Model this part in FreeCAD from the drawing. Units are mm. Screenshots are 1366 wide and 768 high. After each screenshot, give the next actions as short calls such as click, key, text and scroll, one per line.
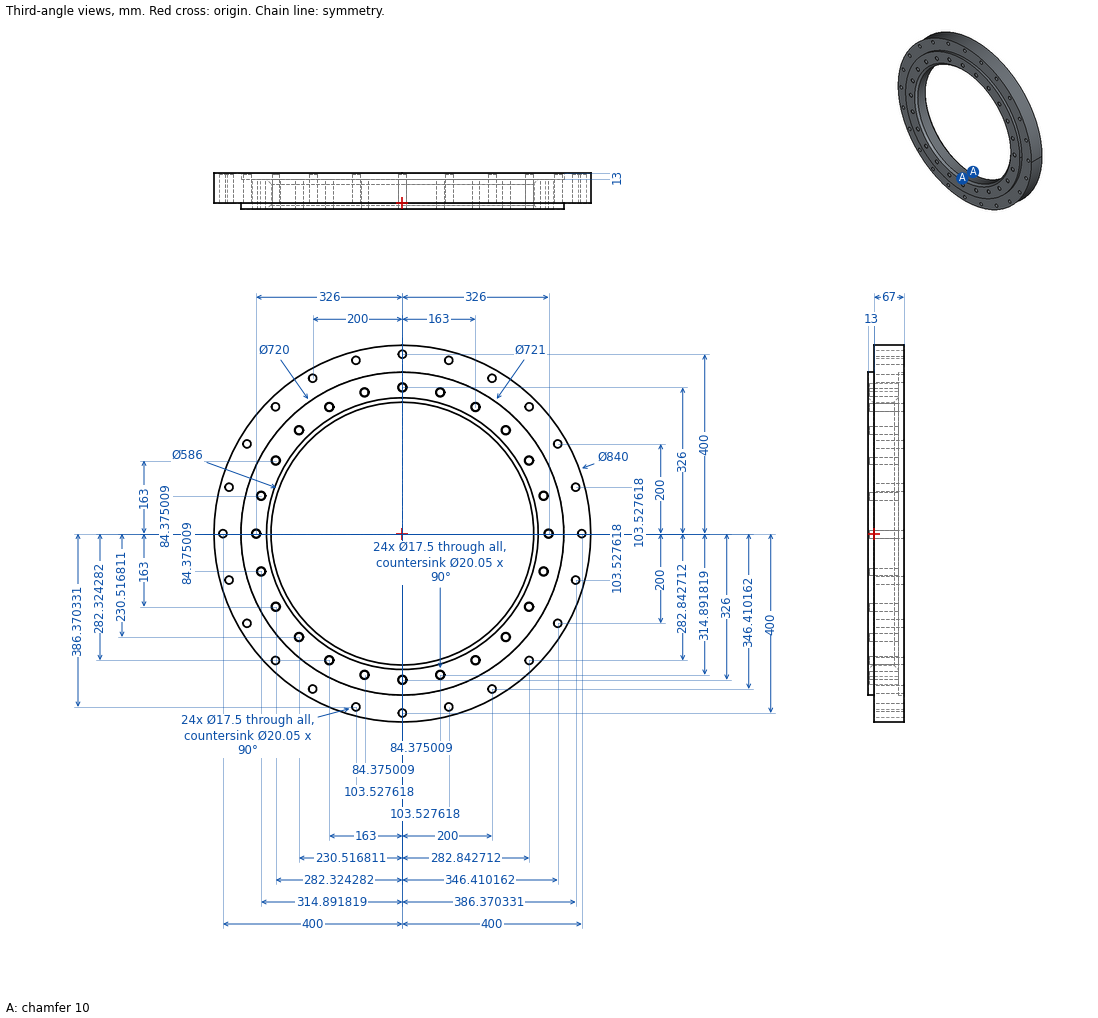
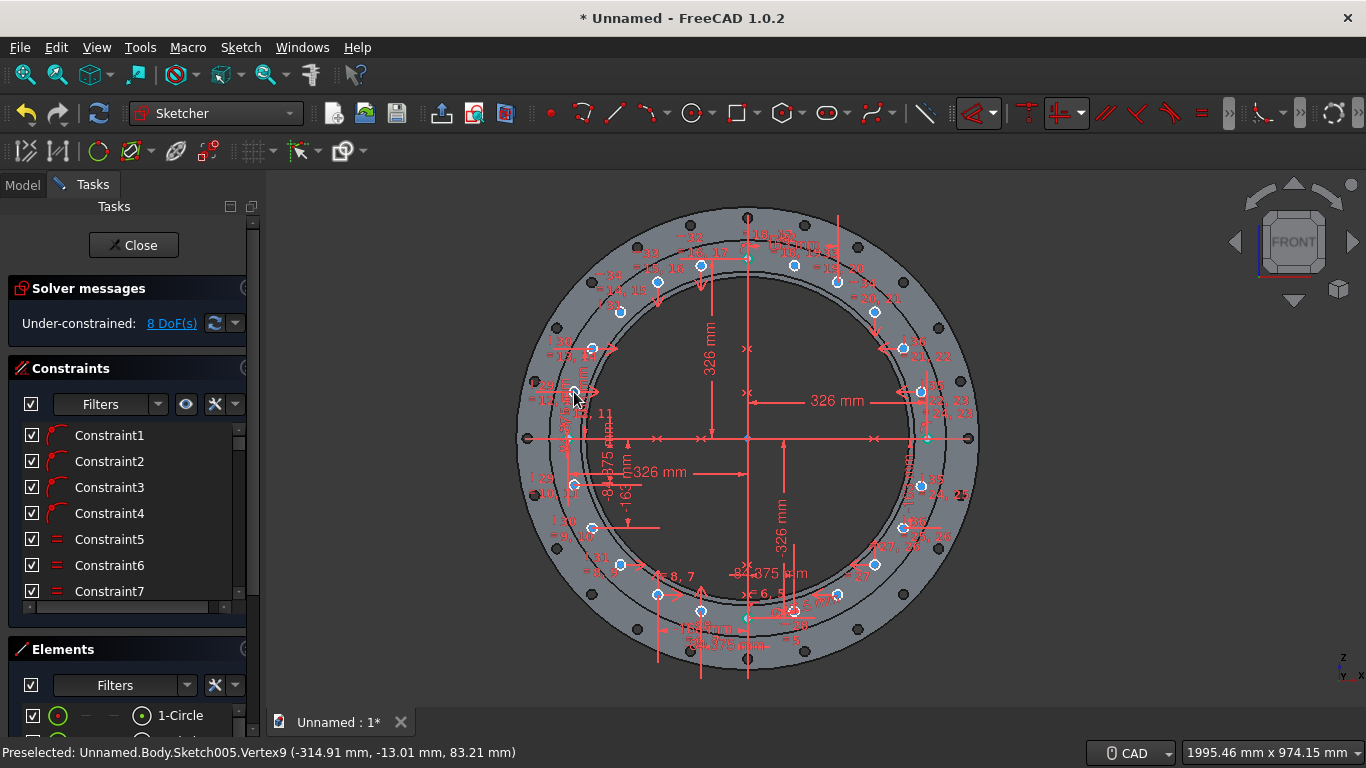
click(795, 266)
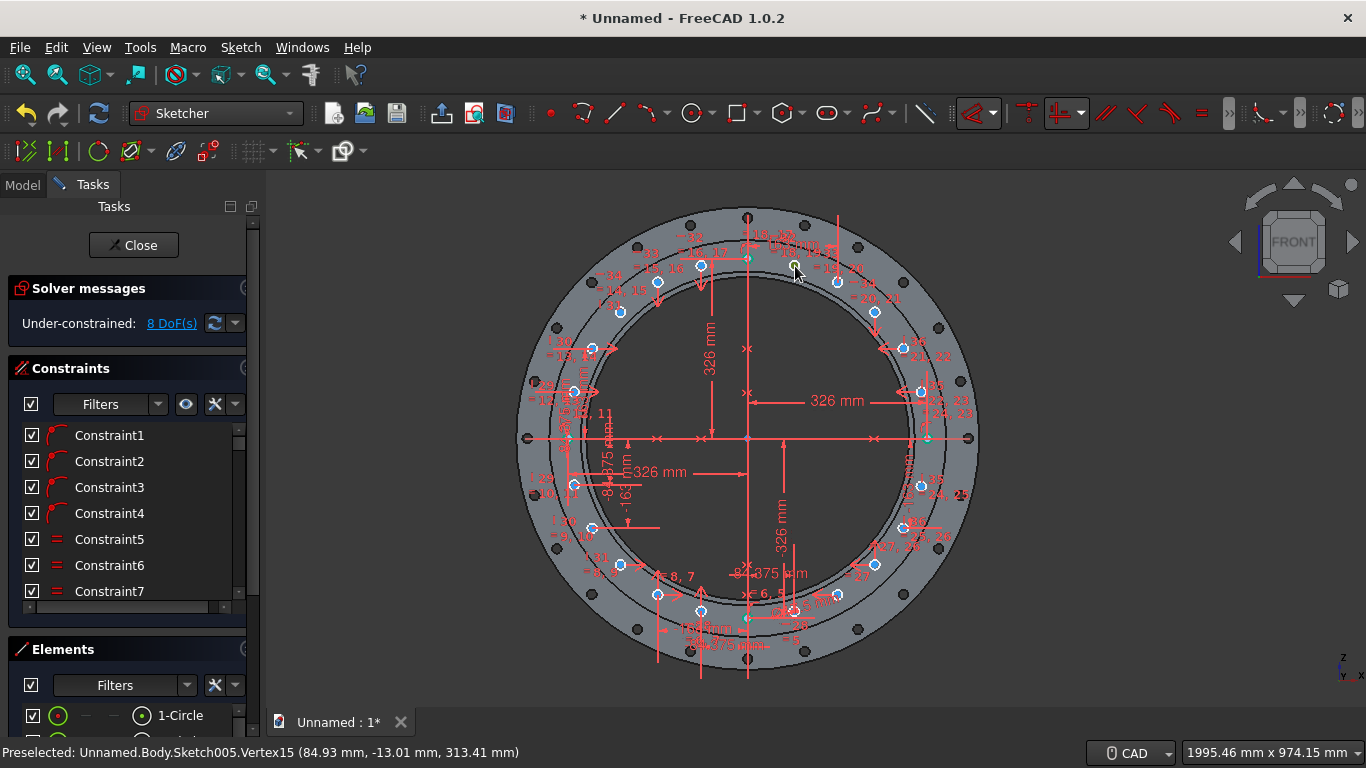
click(996, 114)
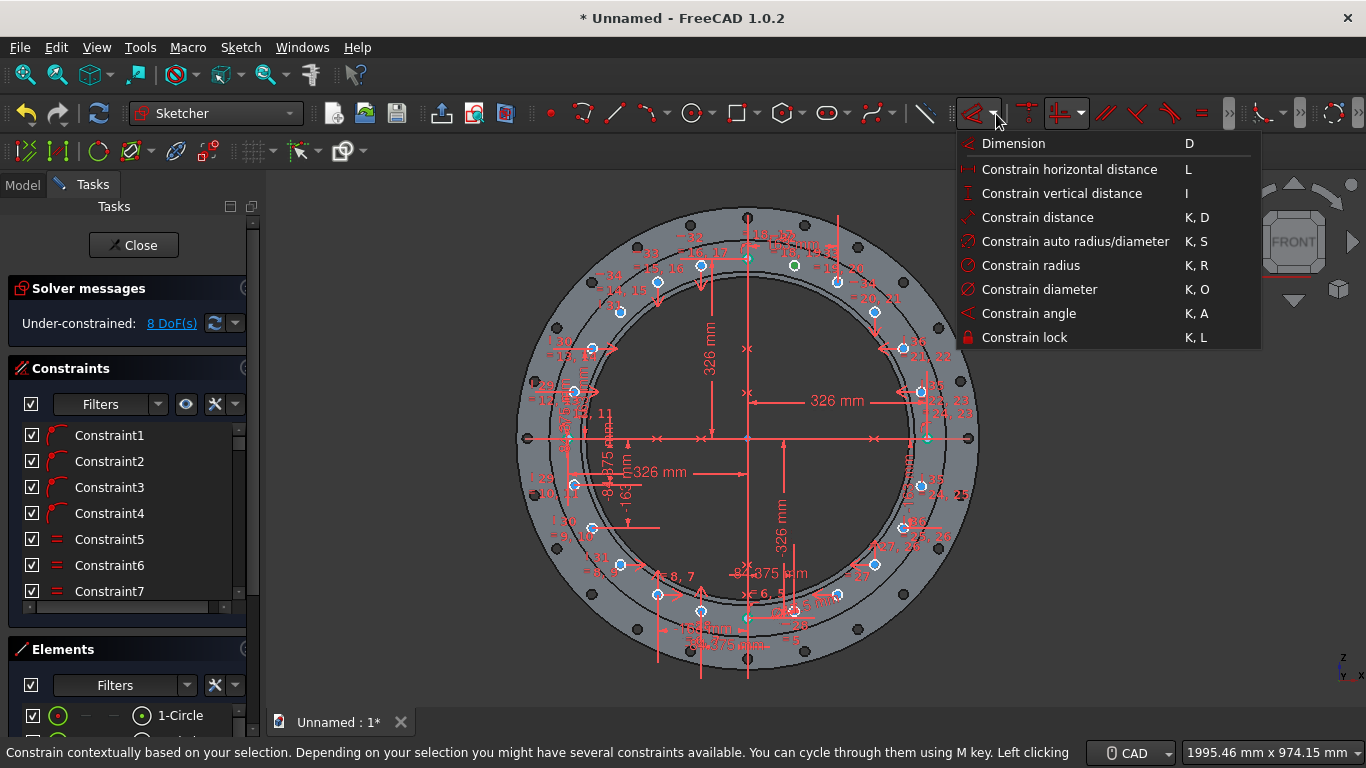
click(1109, 169)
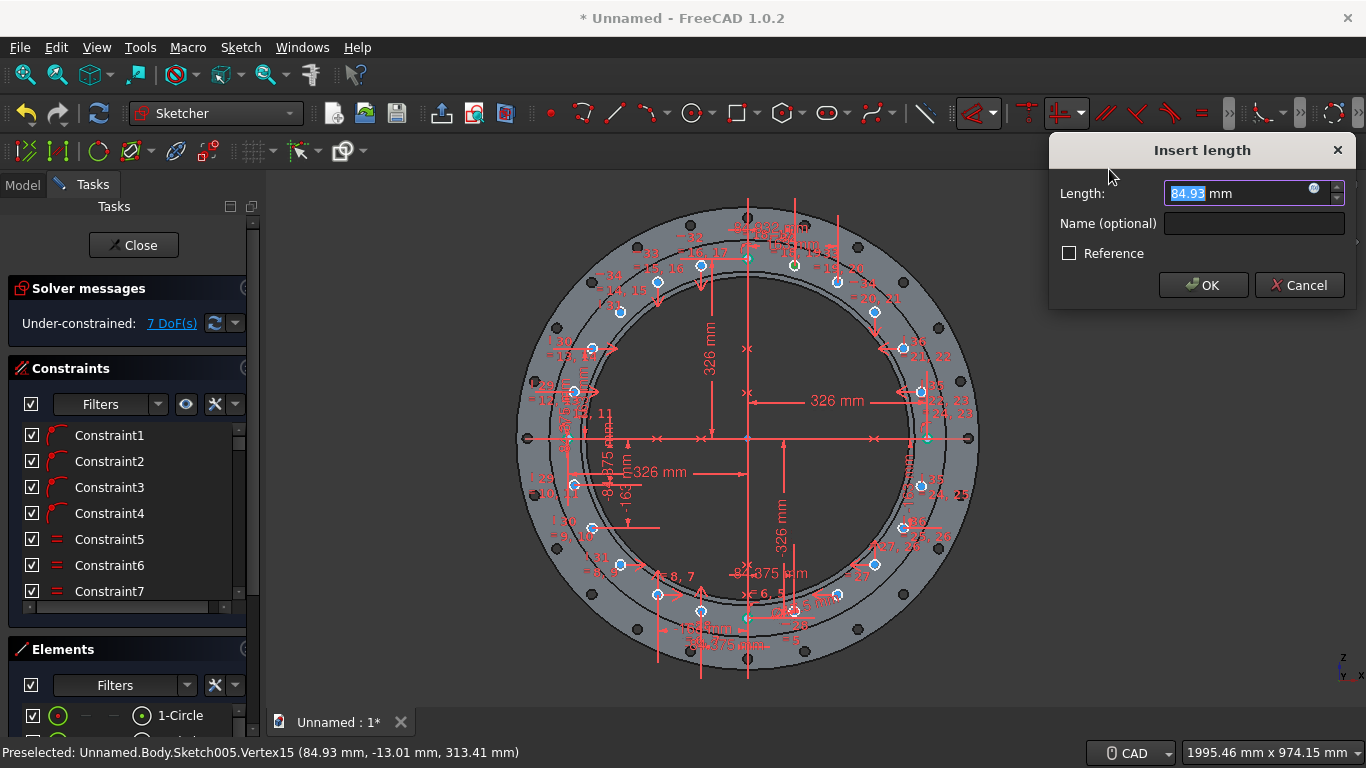
text(84.375009)
key(Return)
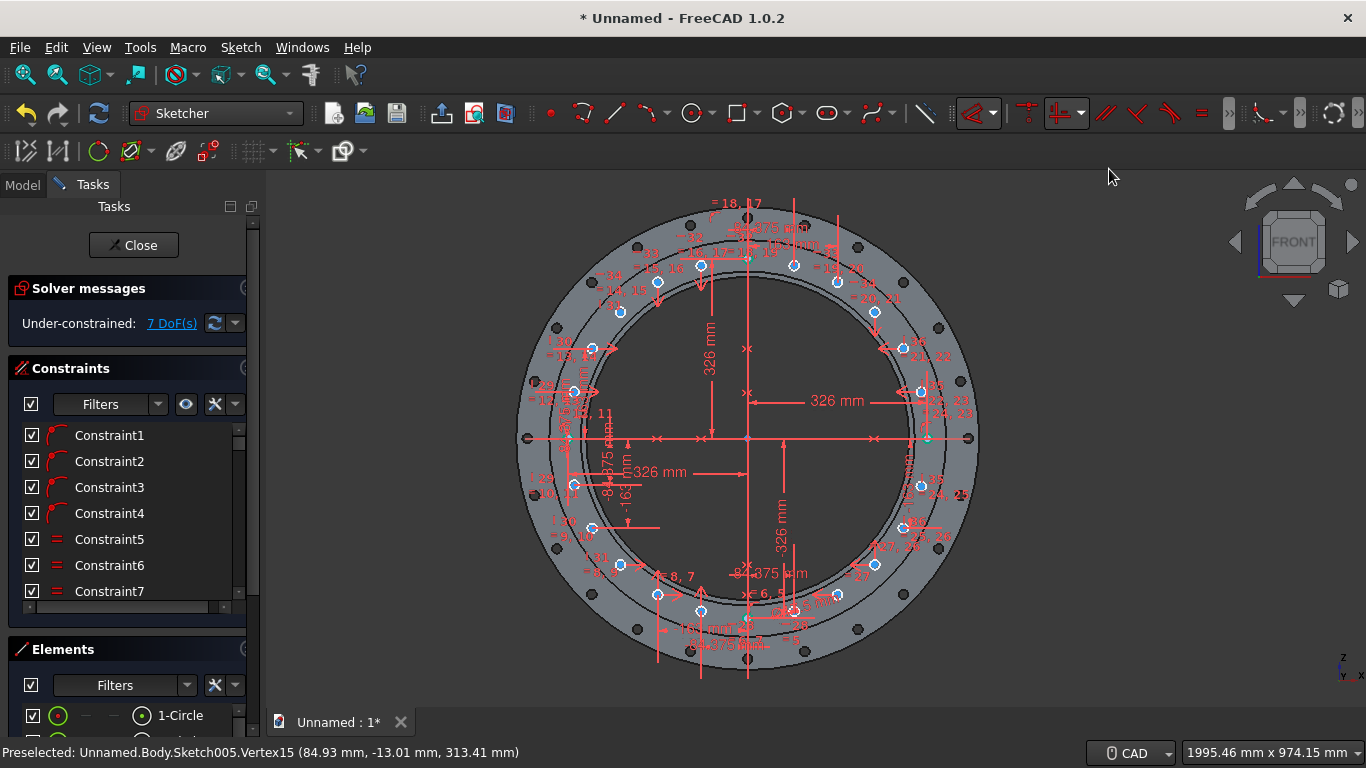
scroll(921, 486, up, 4)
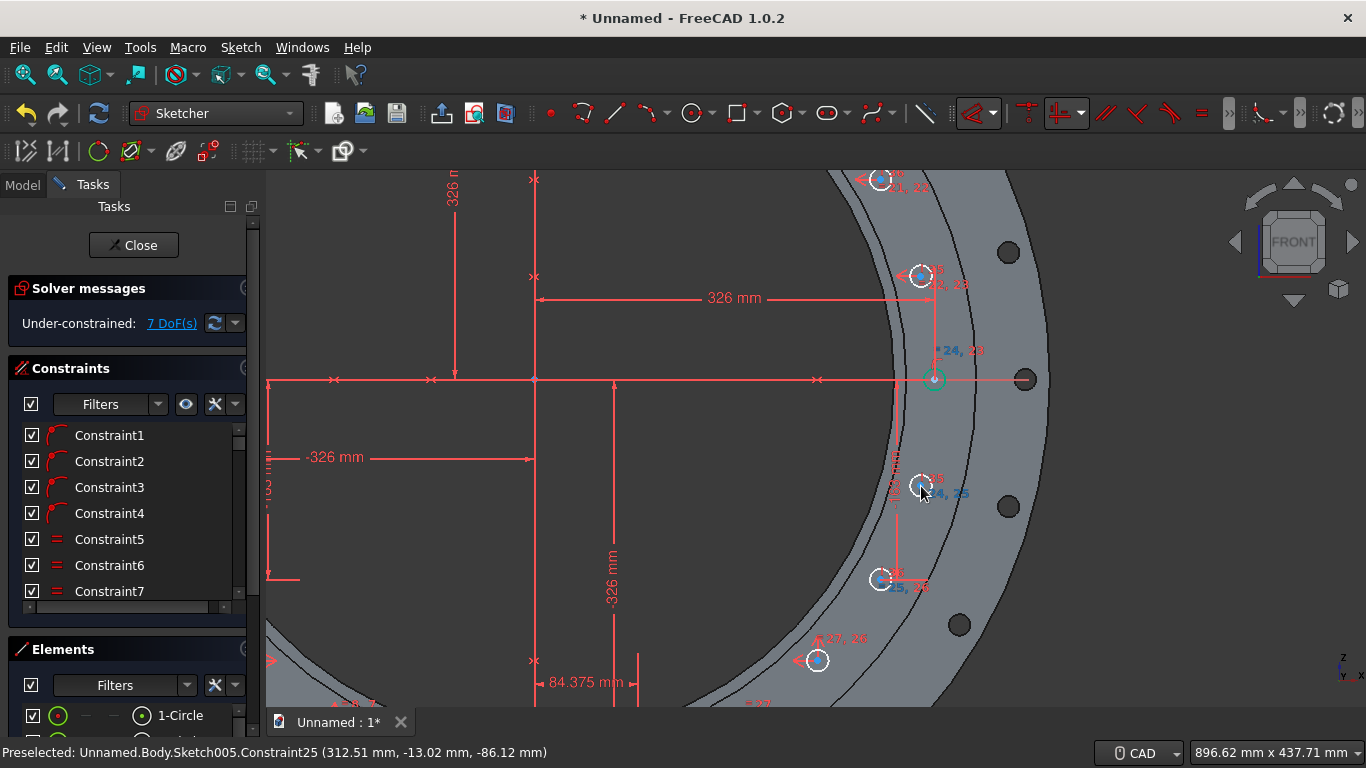
scroll(921, 486, up, 4)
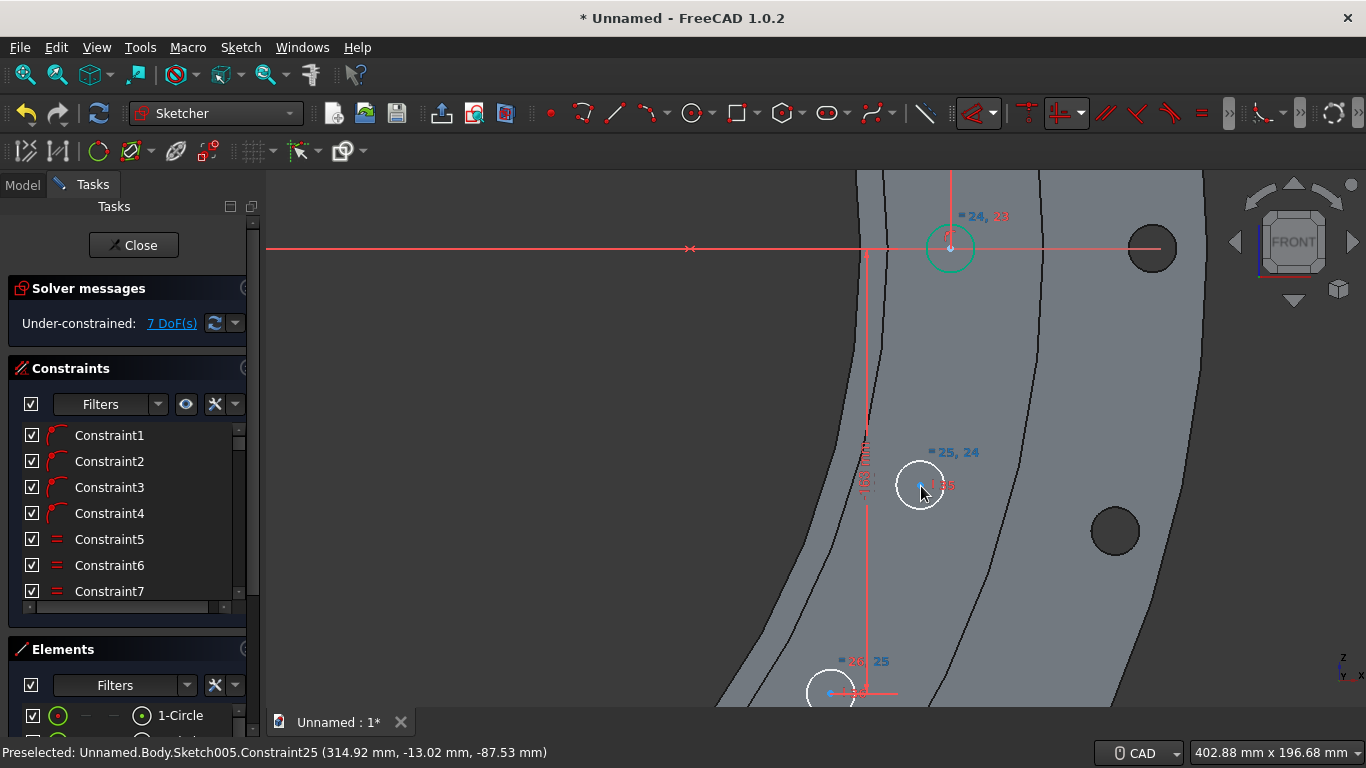
click(920, 485)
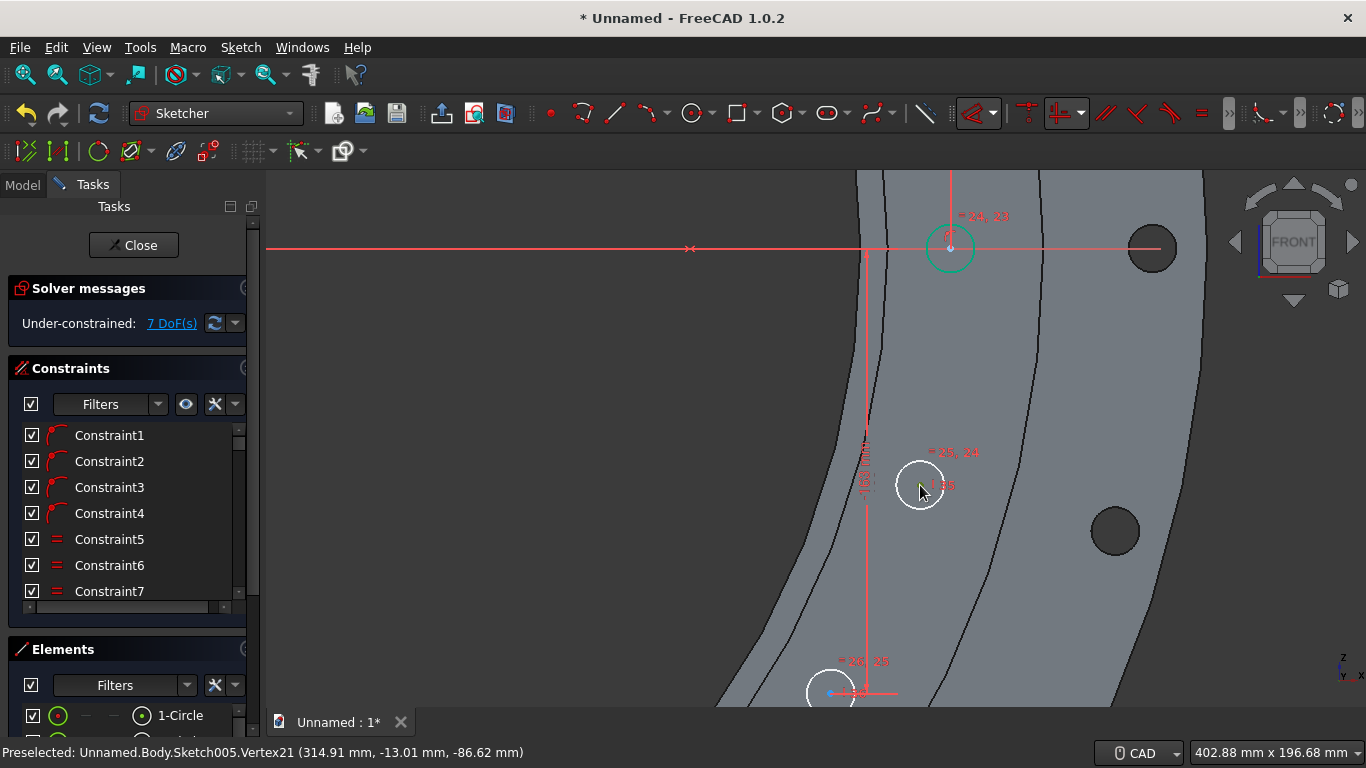
key(i)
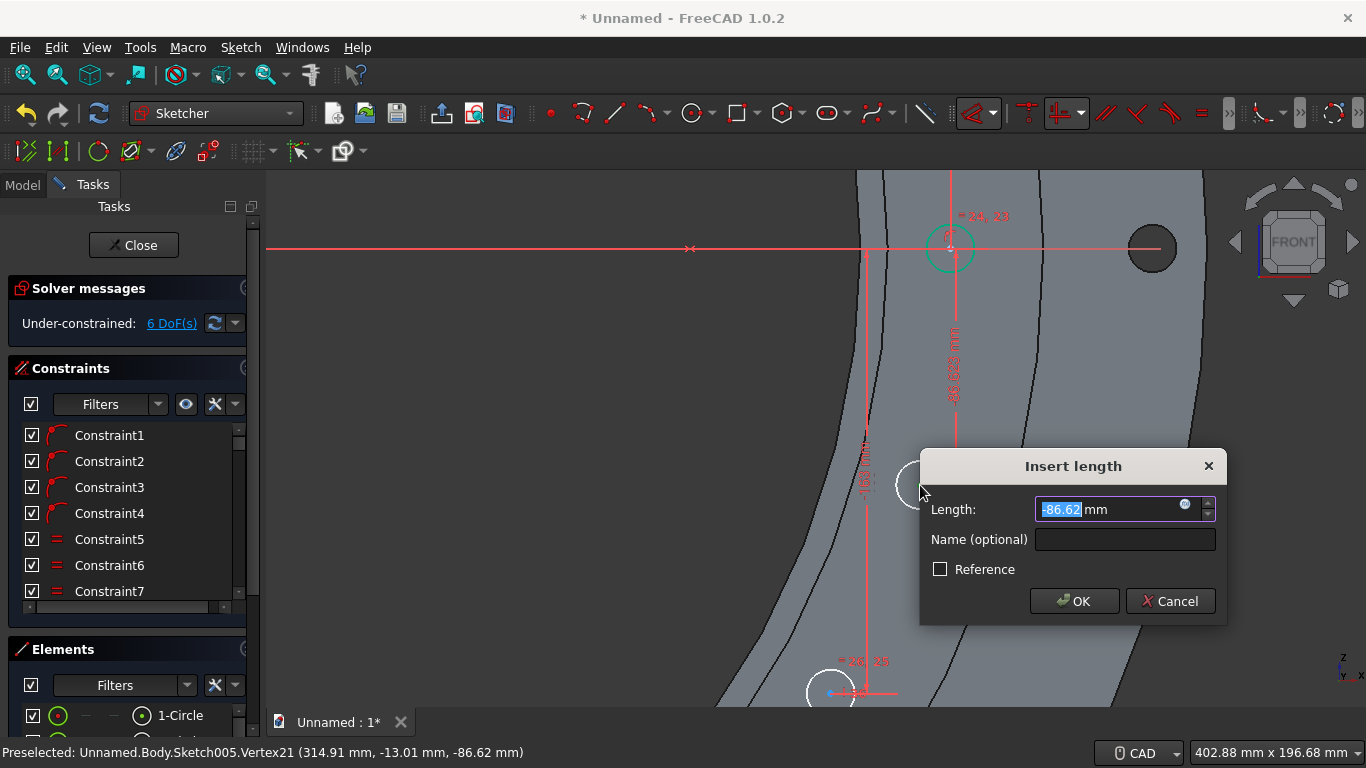
text(-84.375009)
key(Return)